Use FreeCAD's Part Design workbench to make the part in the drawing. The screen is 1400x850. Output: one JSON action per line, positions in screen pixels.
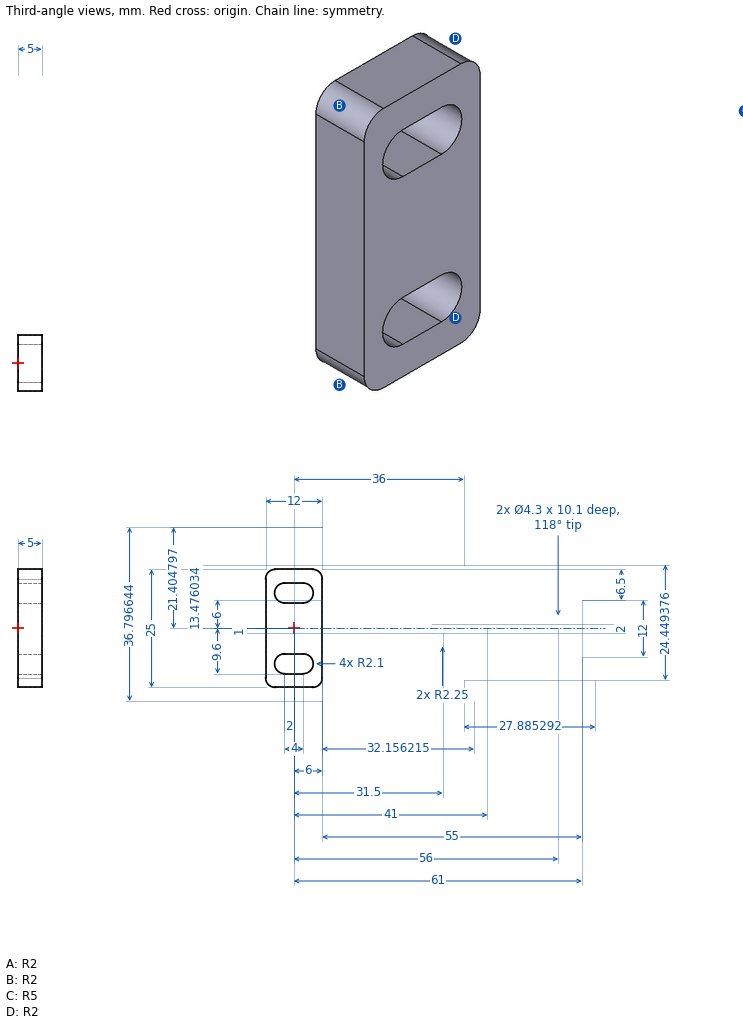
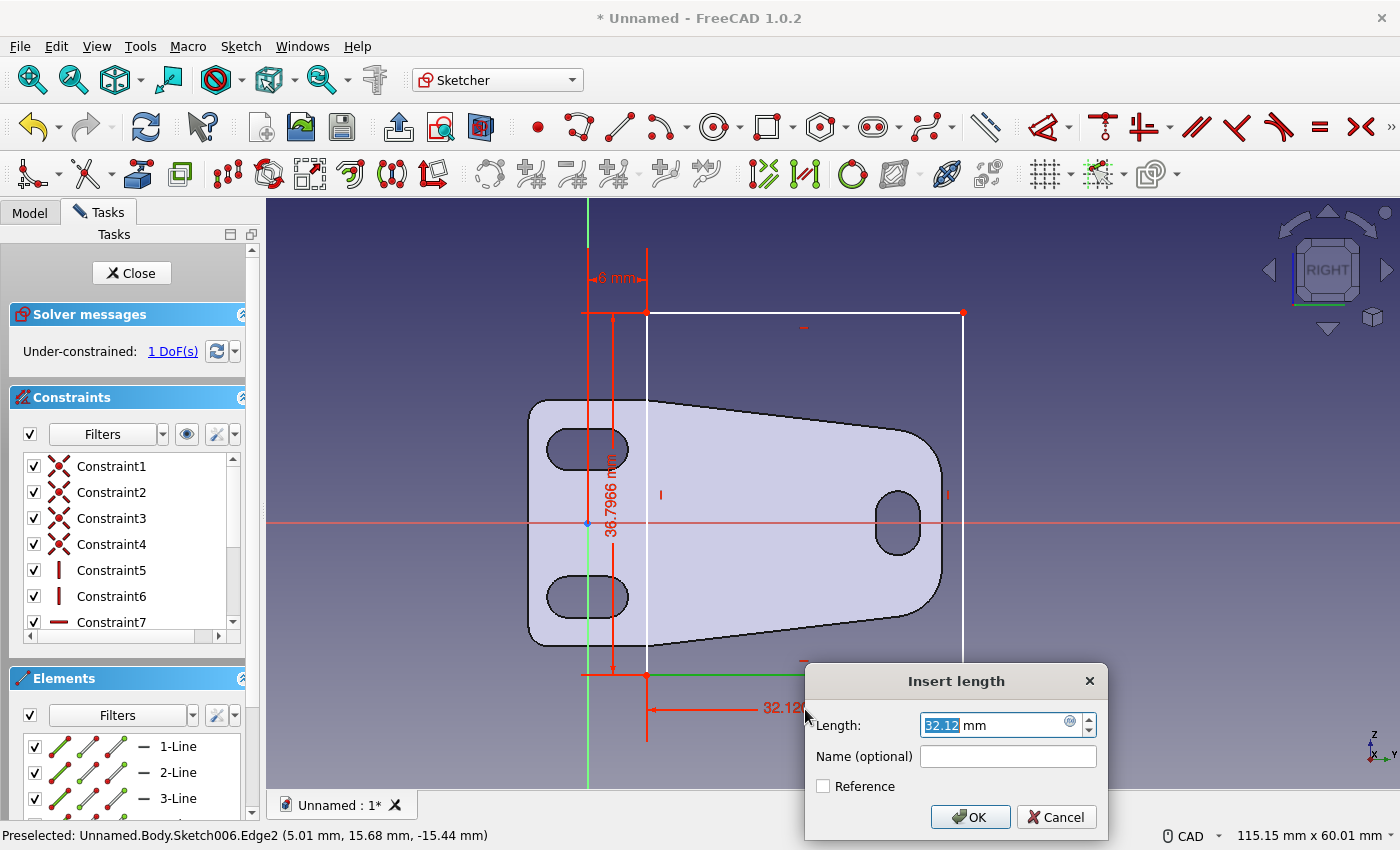
{"action": "type", "text": "32.156215"}
{"action": "key", "text": "Return"}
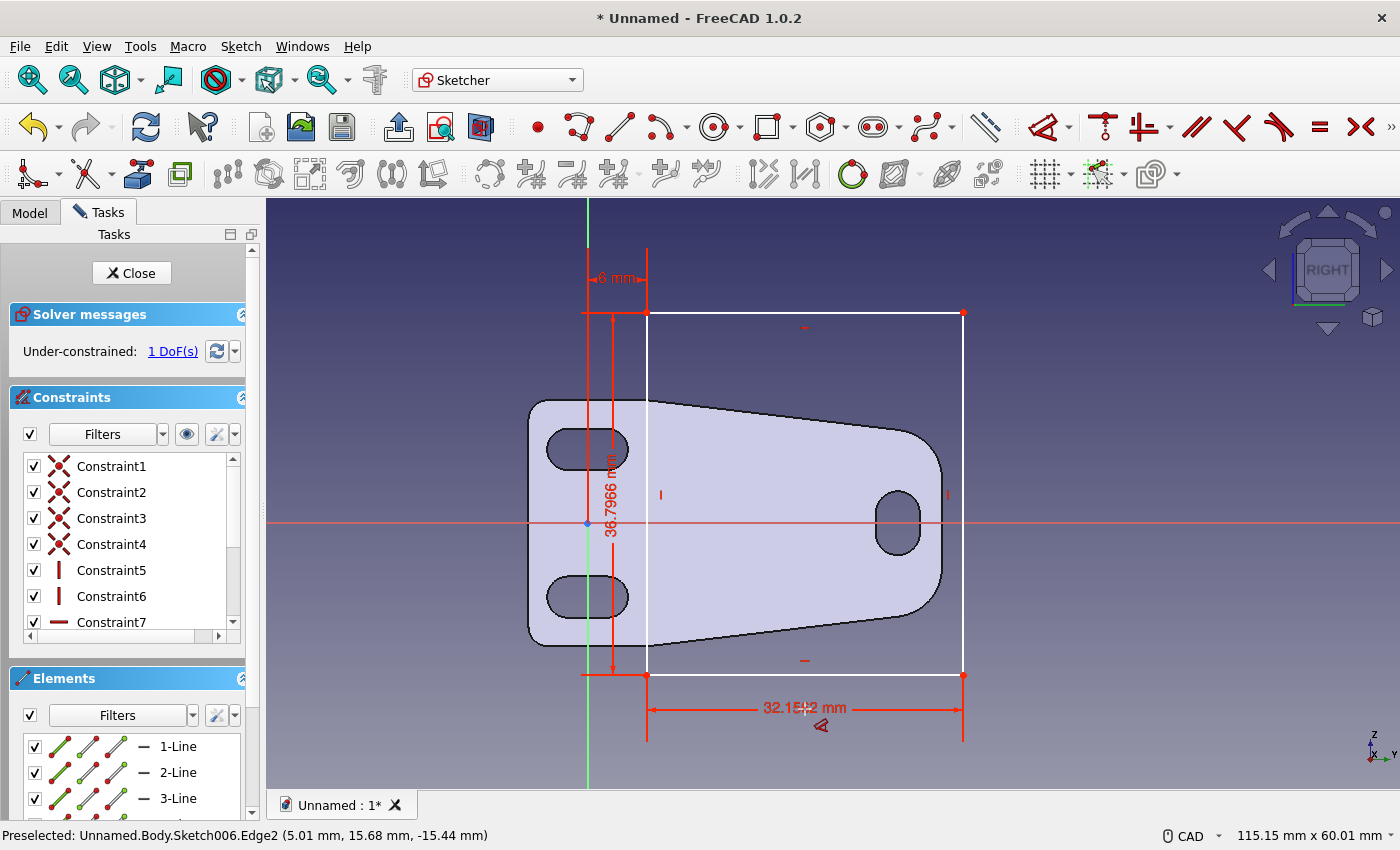
{"action": "left_click", "coordinate": [647, 313]}
{"action": "left_click", "coordinate": [554, 418]}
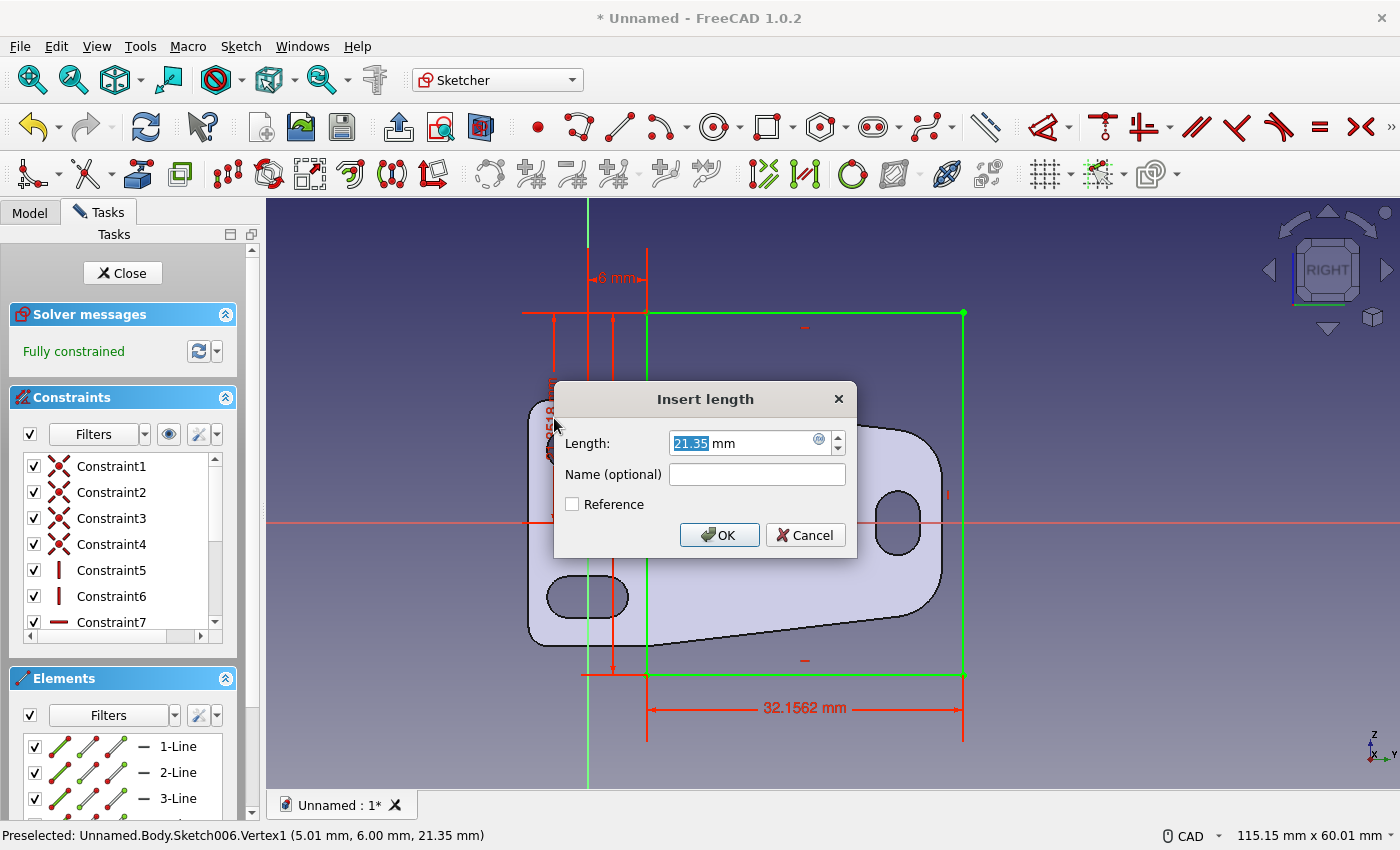
{"action": "type", "text": "21.404797"}
{"action": "key", "text": "Return"}
{"action": "key", "text": "Escape"}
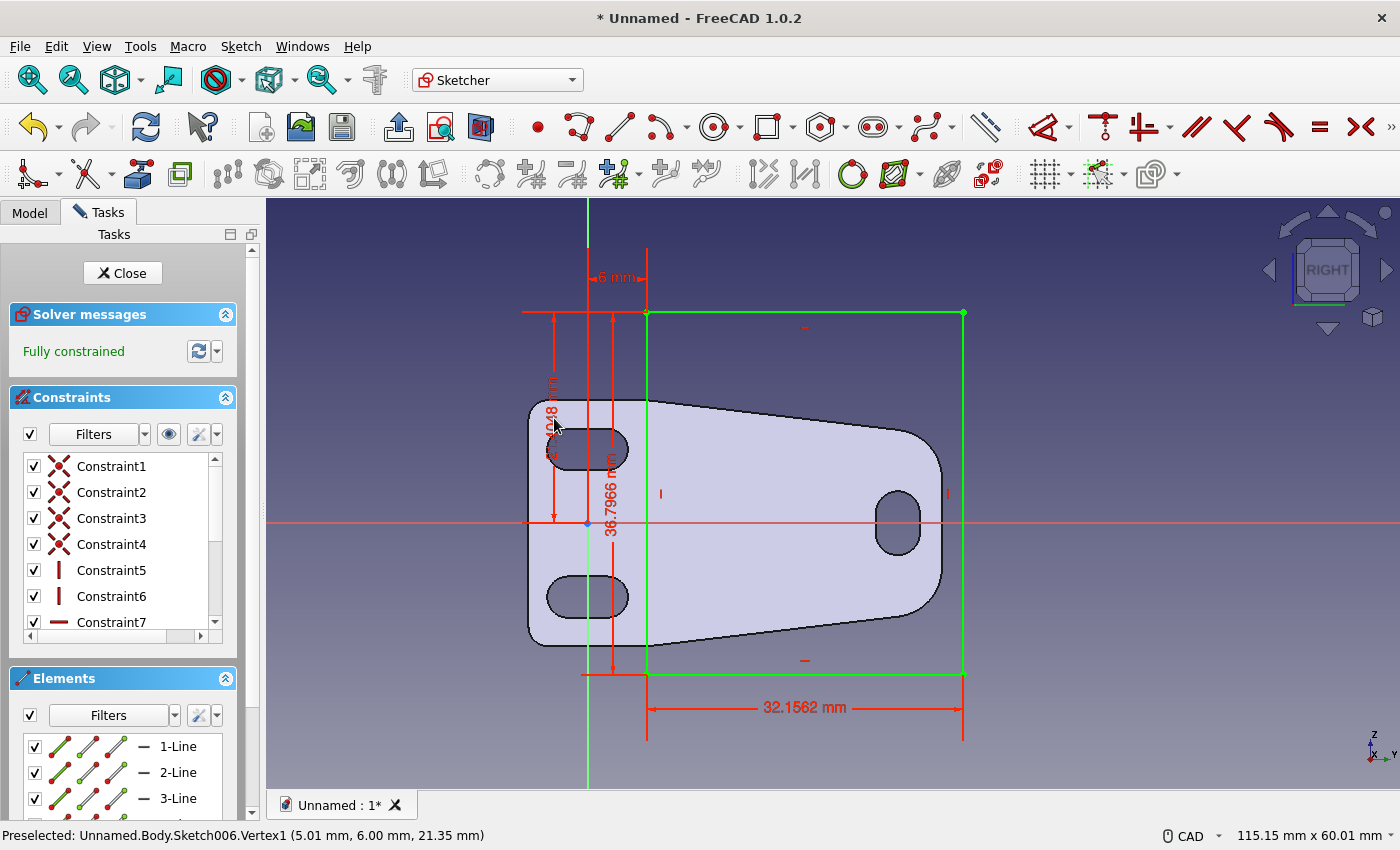
{"action": "left_click", "coordinate": [123, 273]}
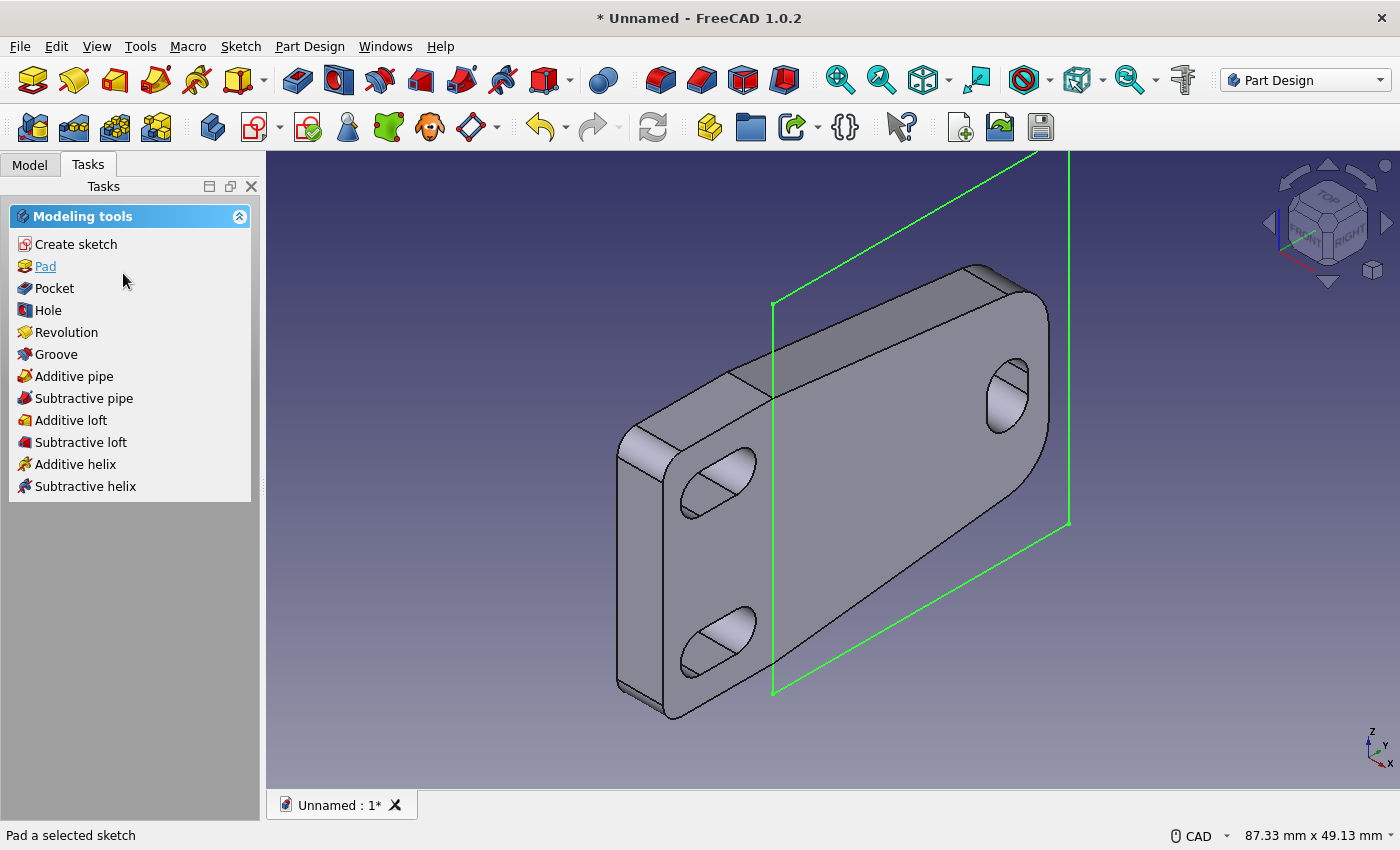
{"action": "left_click", "coordinate": [298, 80]}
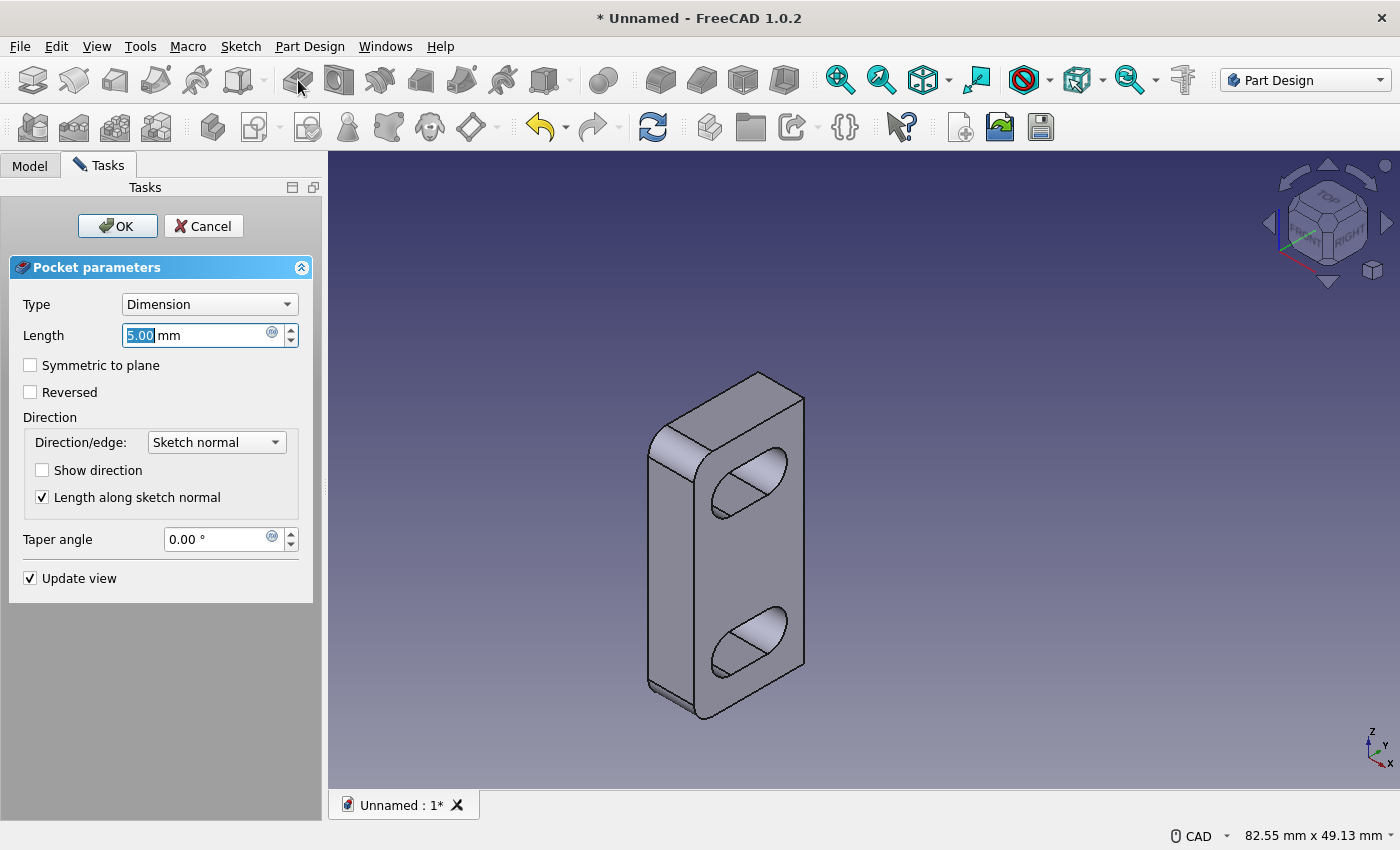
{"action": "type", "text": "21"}
{"action": "key", "text": "Tab"}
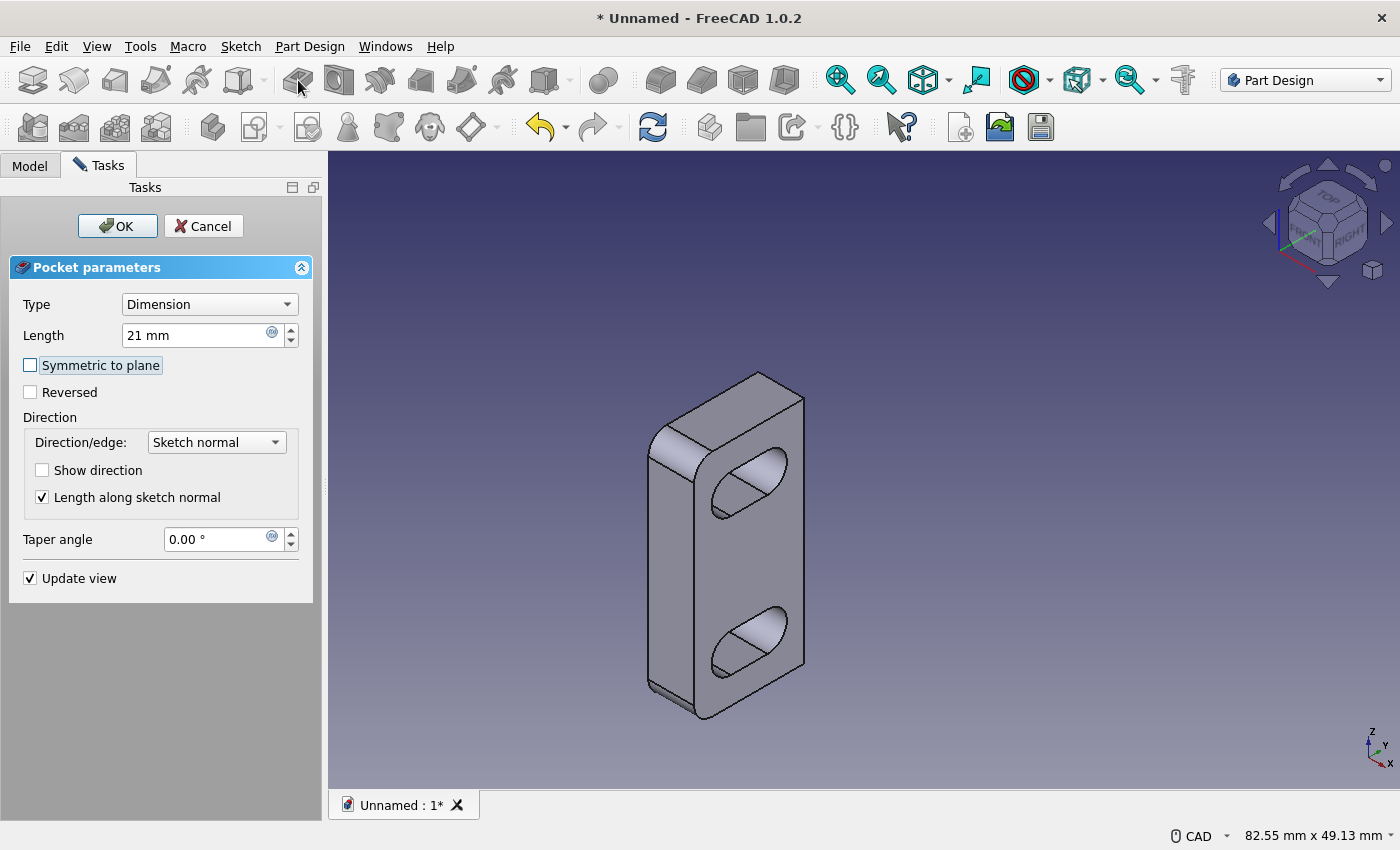
{"action": "left_click", "coordinate": [118, 226]}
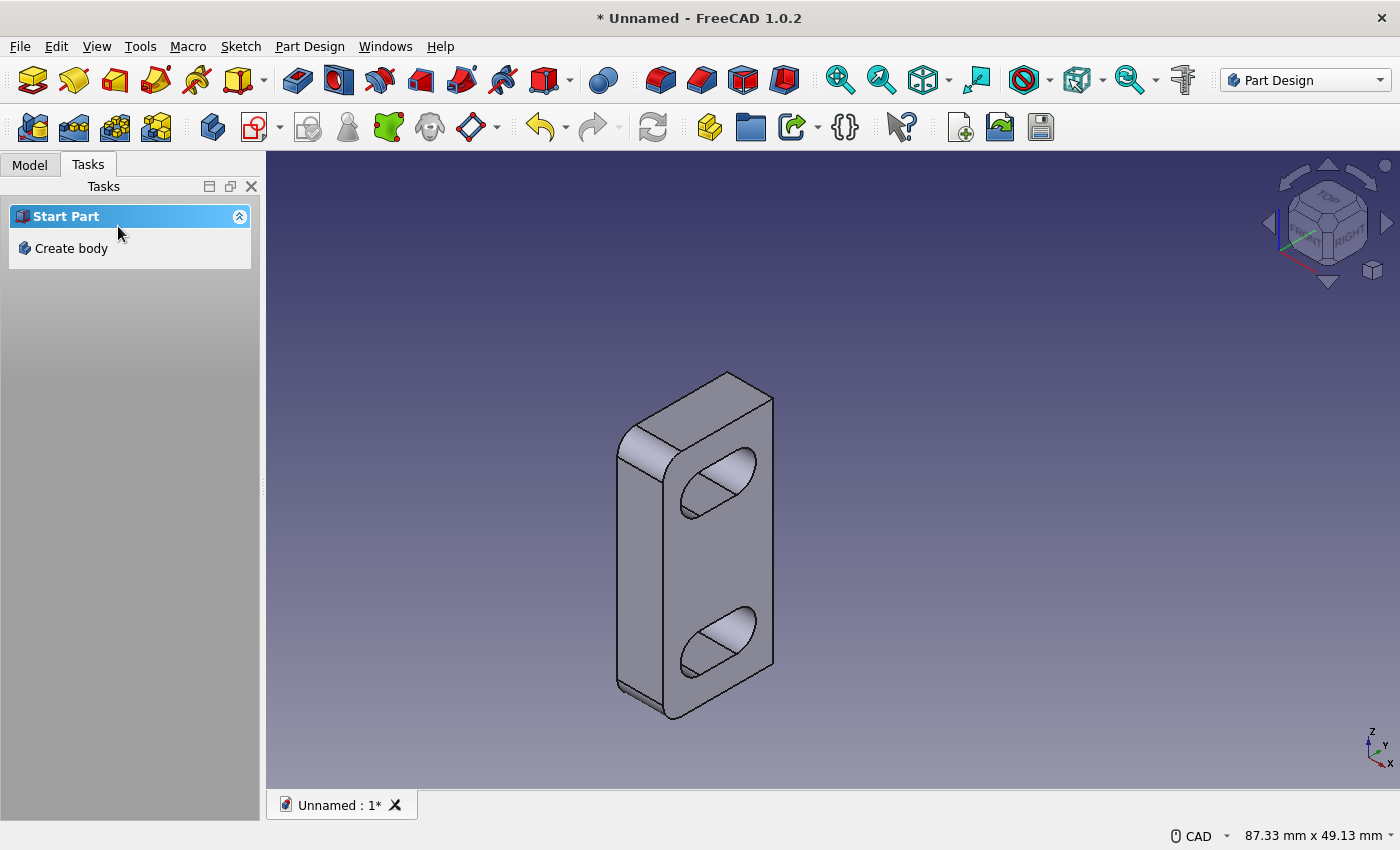
{"action": "key", "text": "2"}